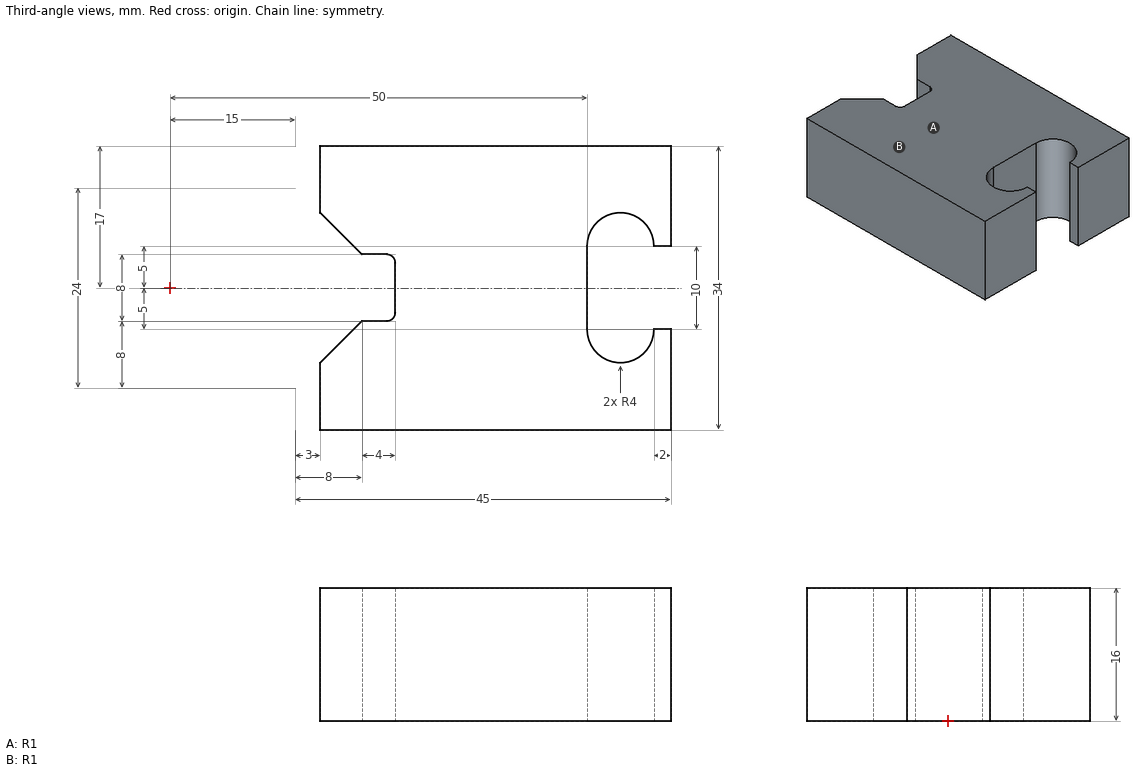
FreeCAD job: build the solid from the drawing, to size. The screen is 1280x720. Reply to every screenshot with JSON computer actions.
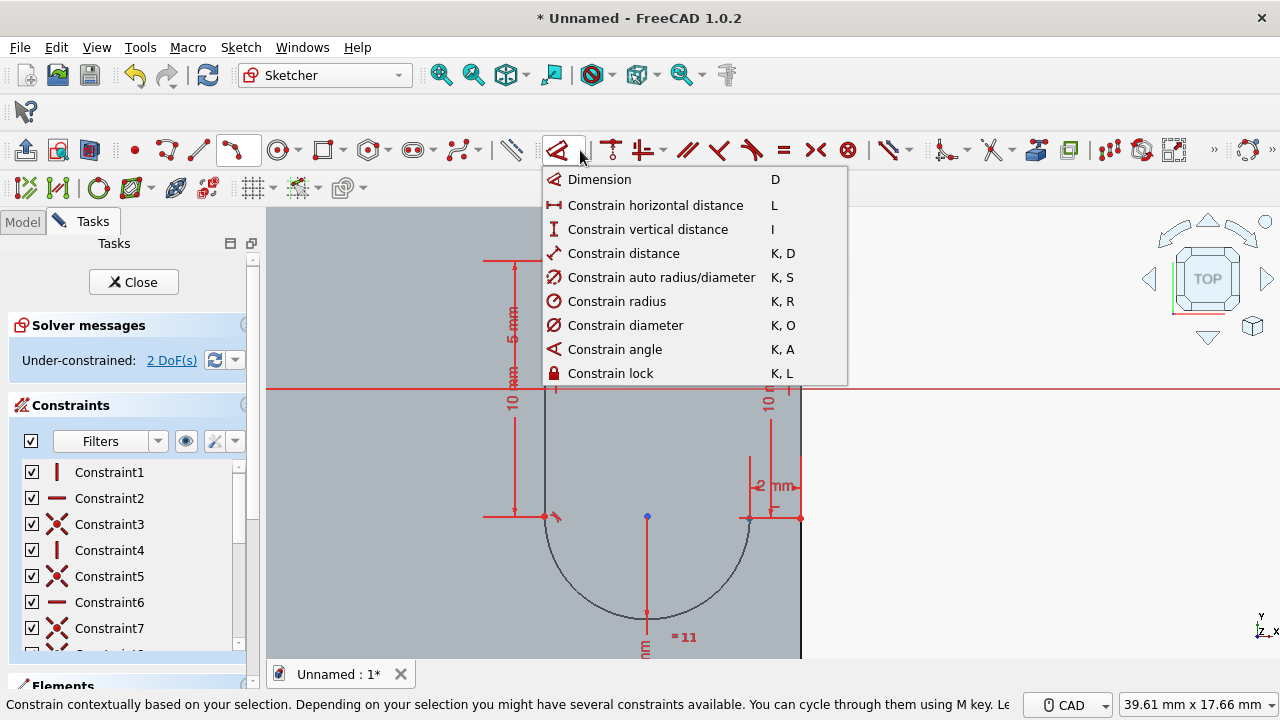
{"action": "left_click", "coordinate": [695, 229]}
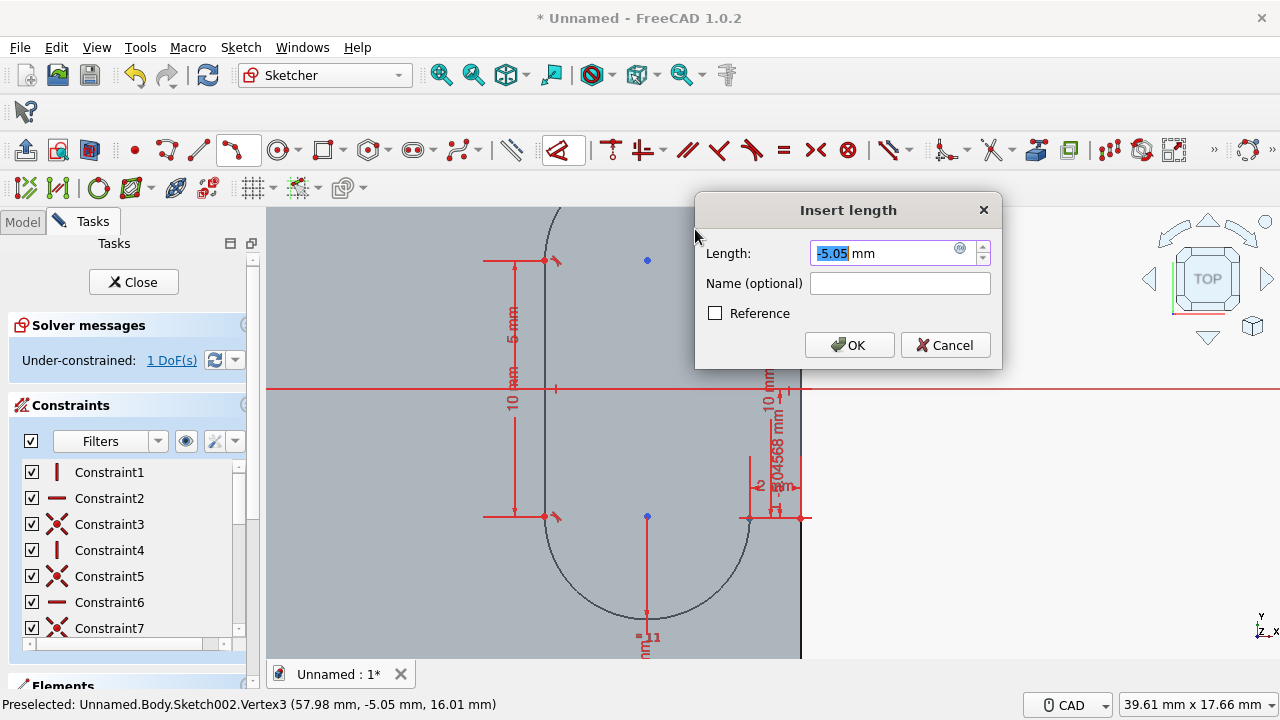
{"action": "type", "text": "-5"}
{"action": "key", "text": "Return"}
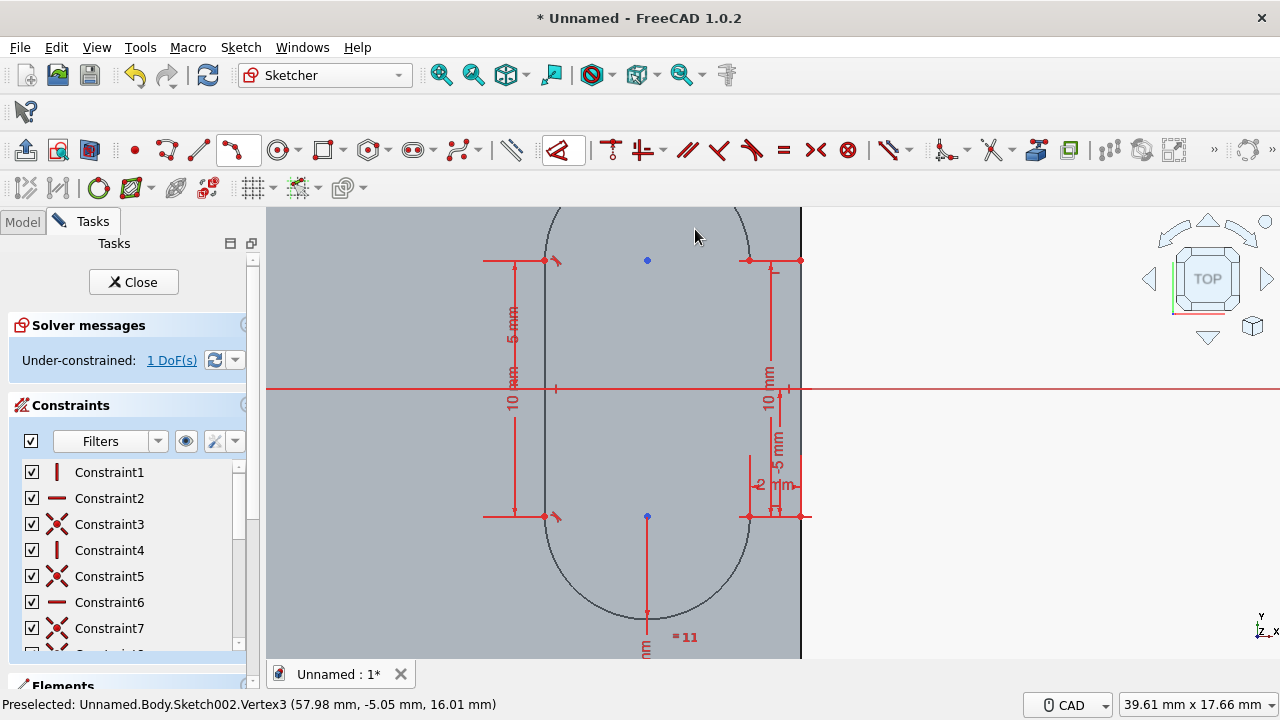
{"action": "left_click", "coordinate": [545, 261]}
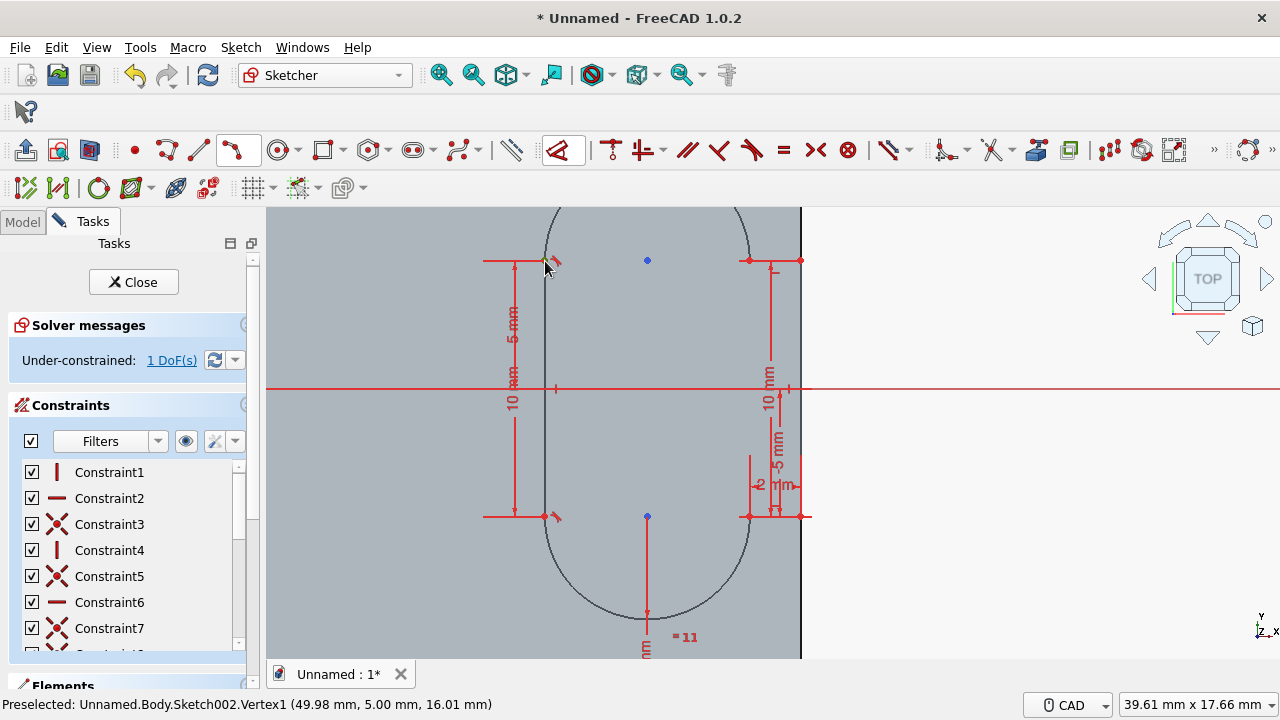
{"action": "key", "text": "l"}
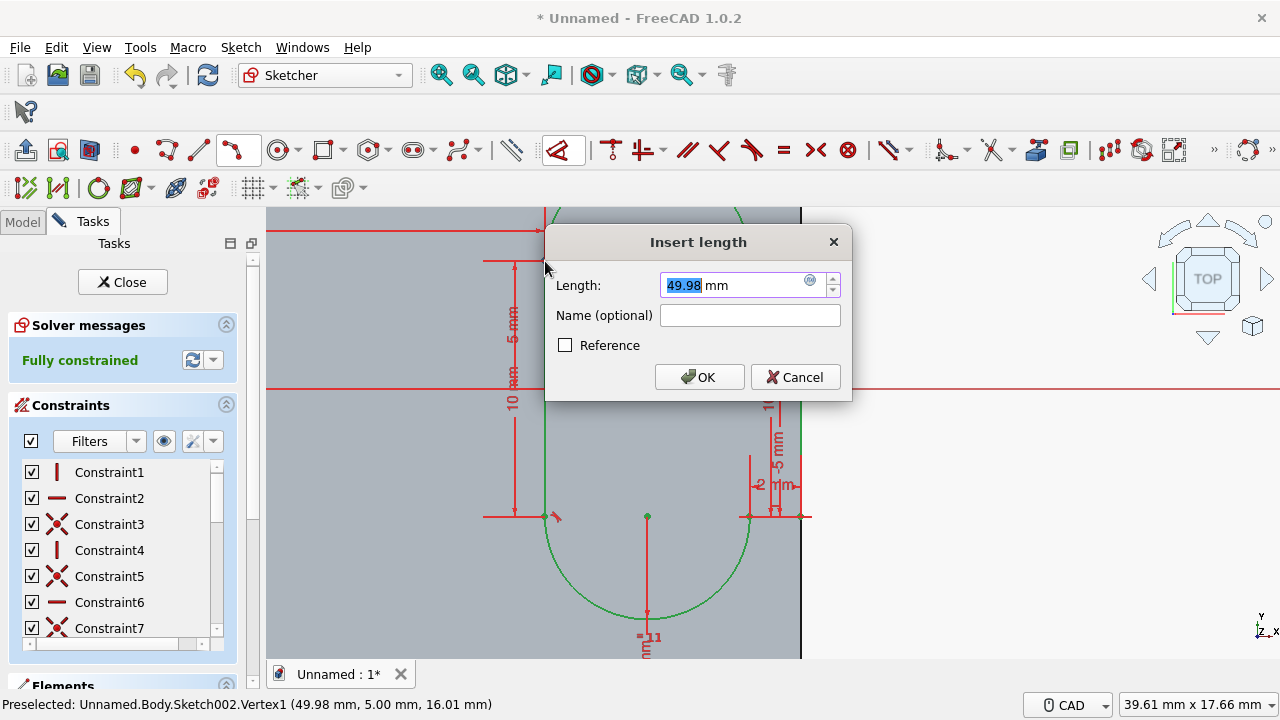
{"action": "type", "text": "50"}
{"action": "key", "text": "Return"}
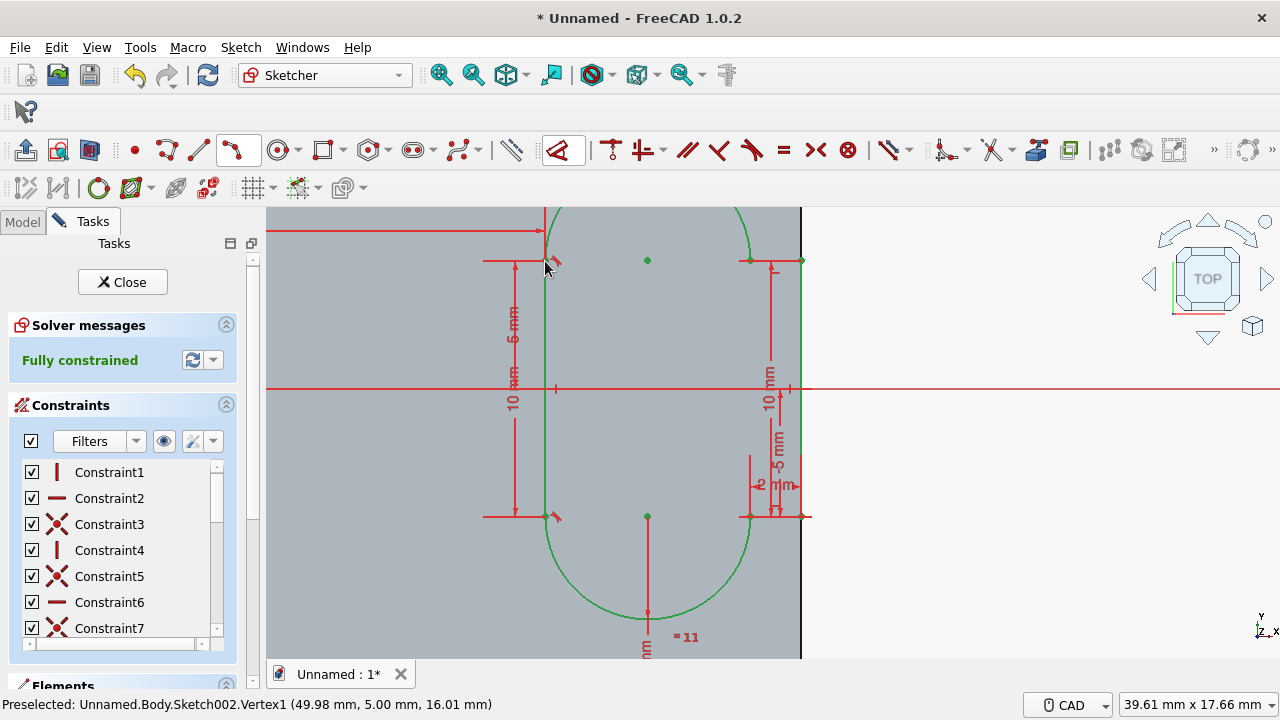
{"action": "left_click", "coordinate": [123, 282]}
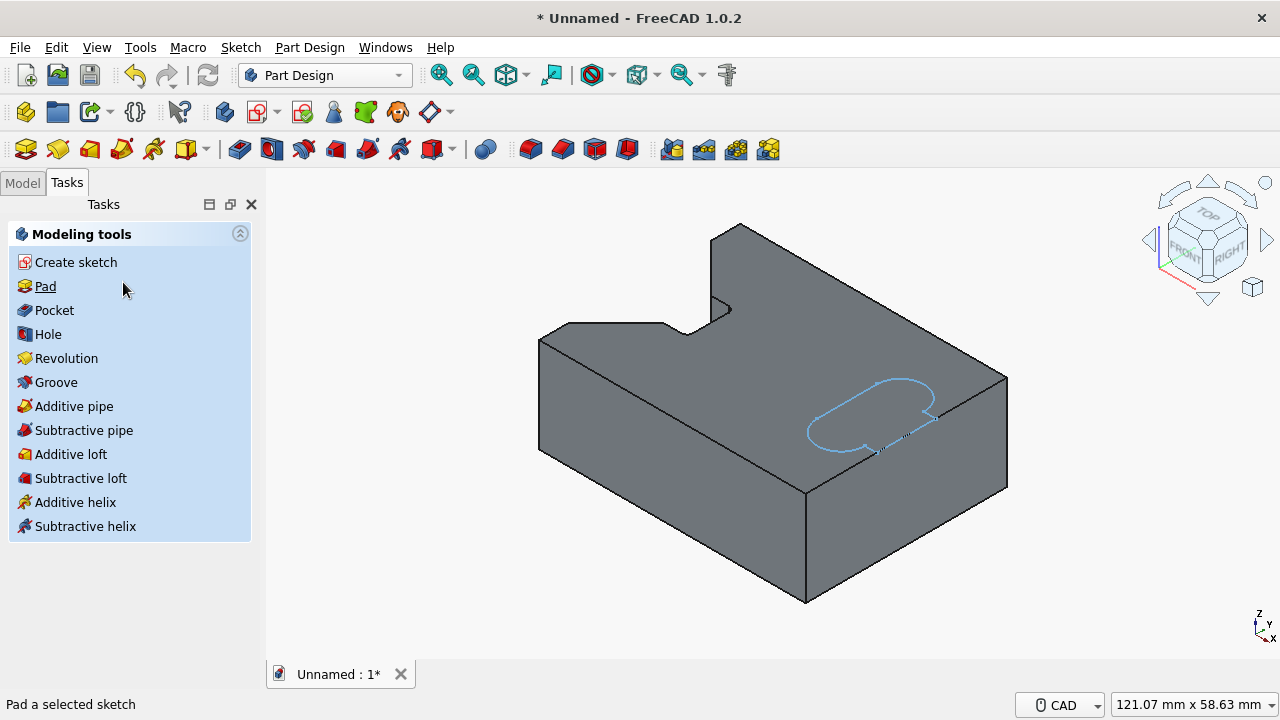
{"action": "left_click", "coordinate": [240, 150]}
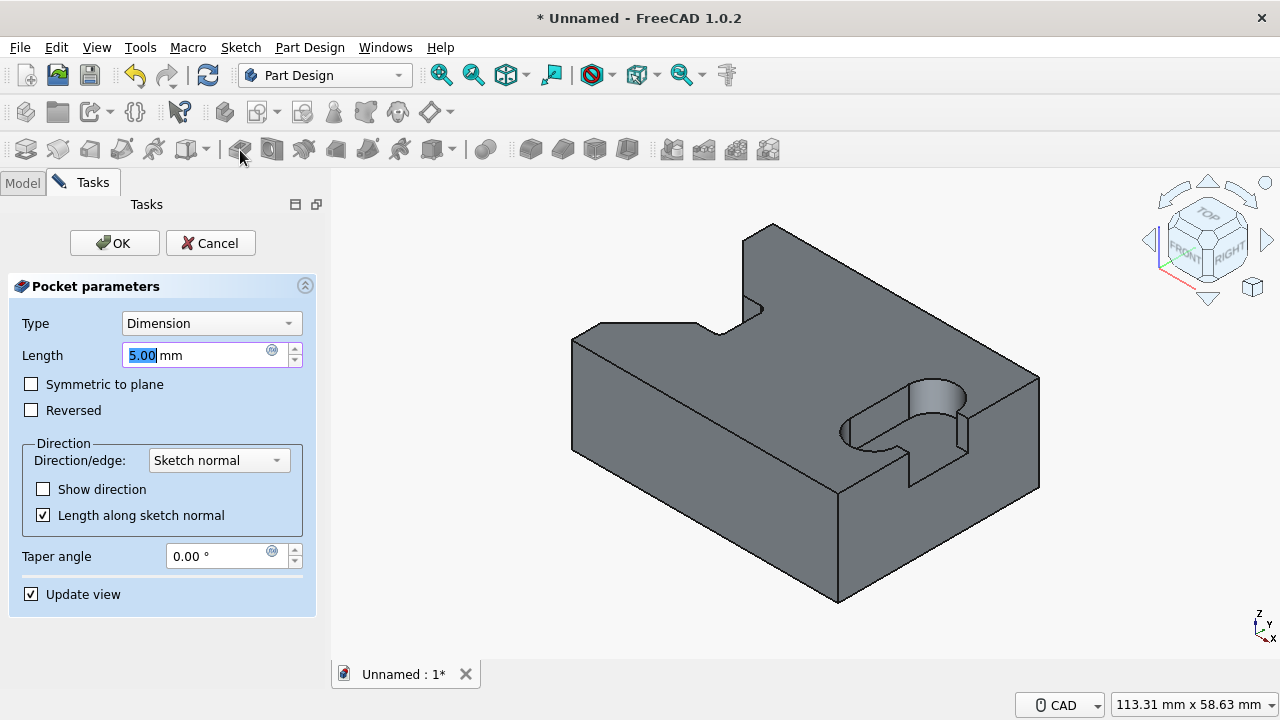
{"action": "left_click", "coordinate": [212, 324]}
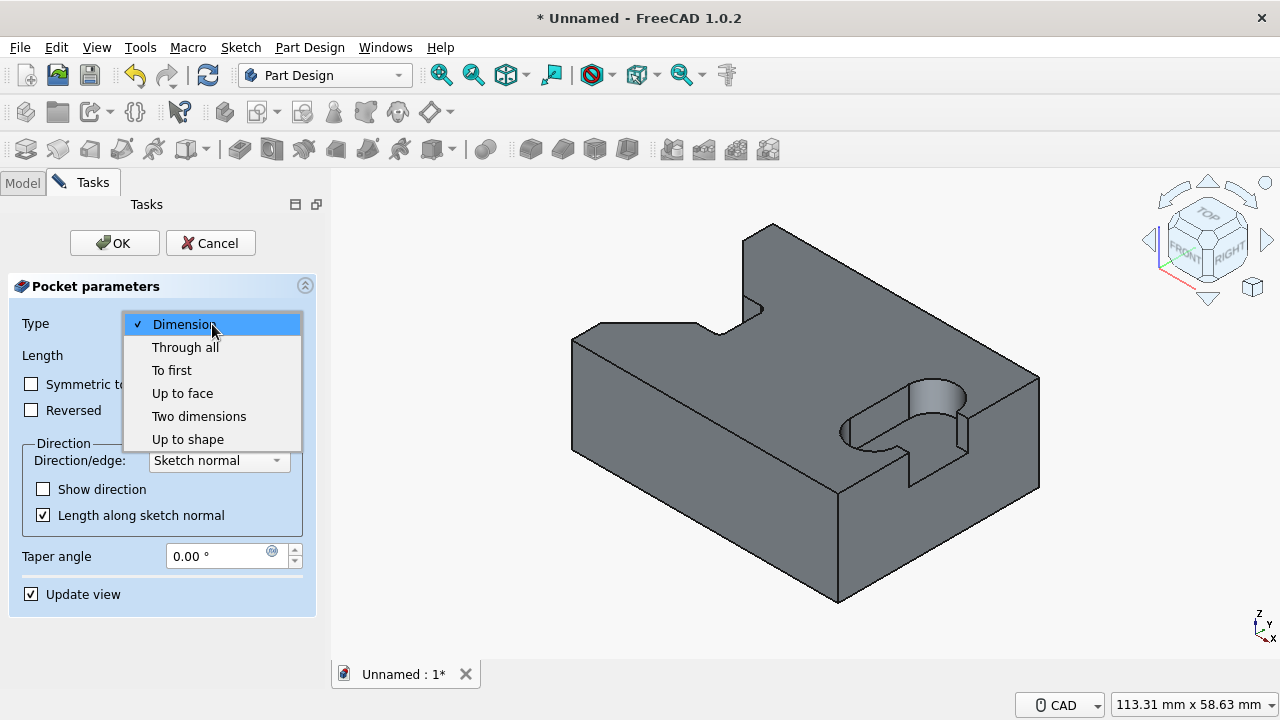
{"action": "left_click", "coordinate": [212, 348]}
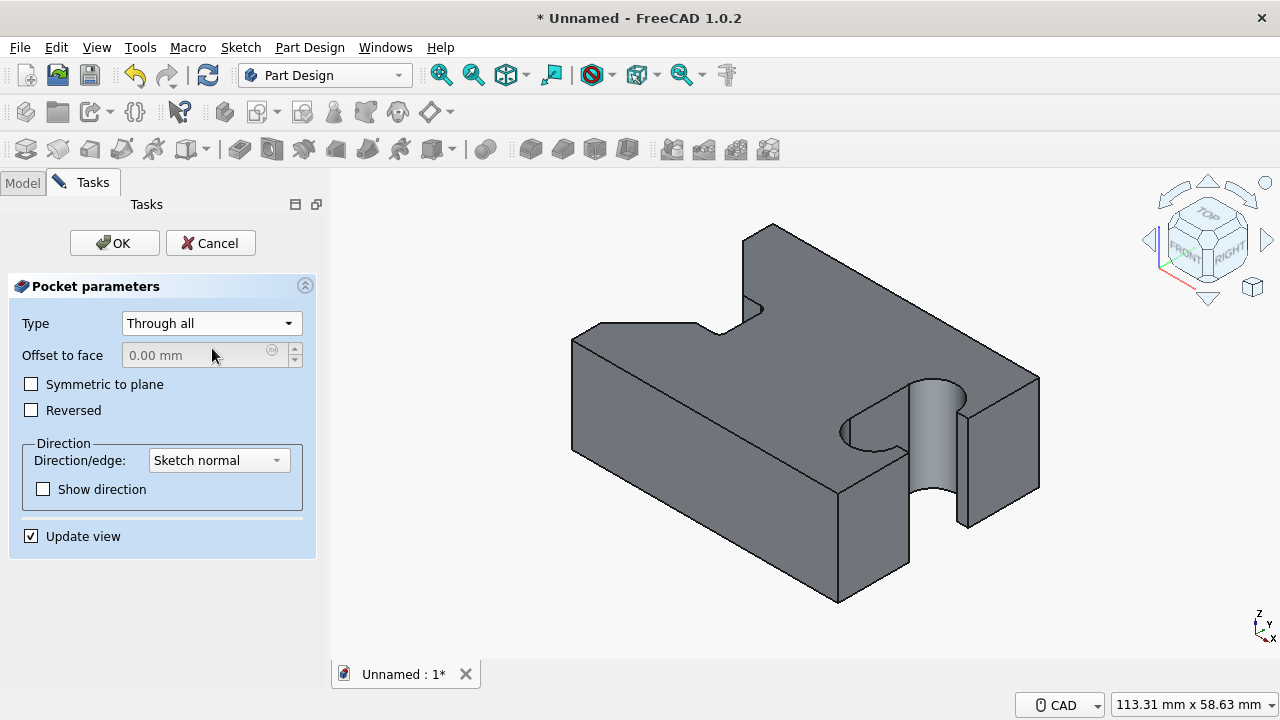
{"action": "left_click", "coordinate": [115, 243]}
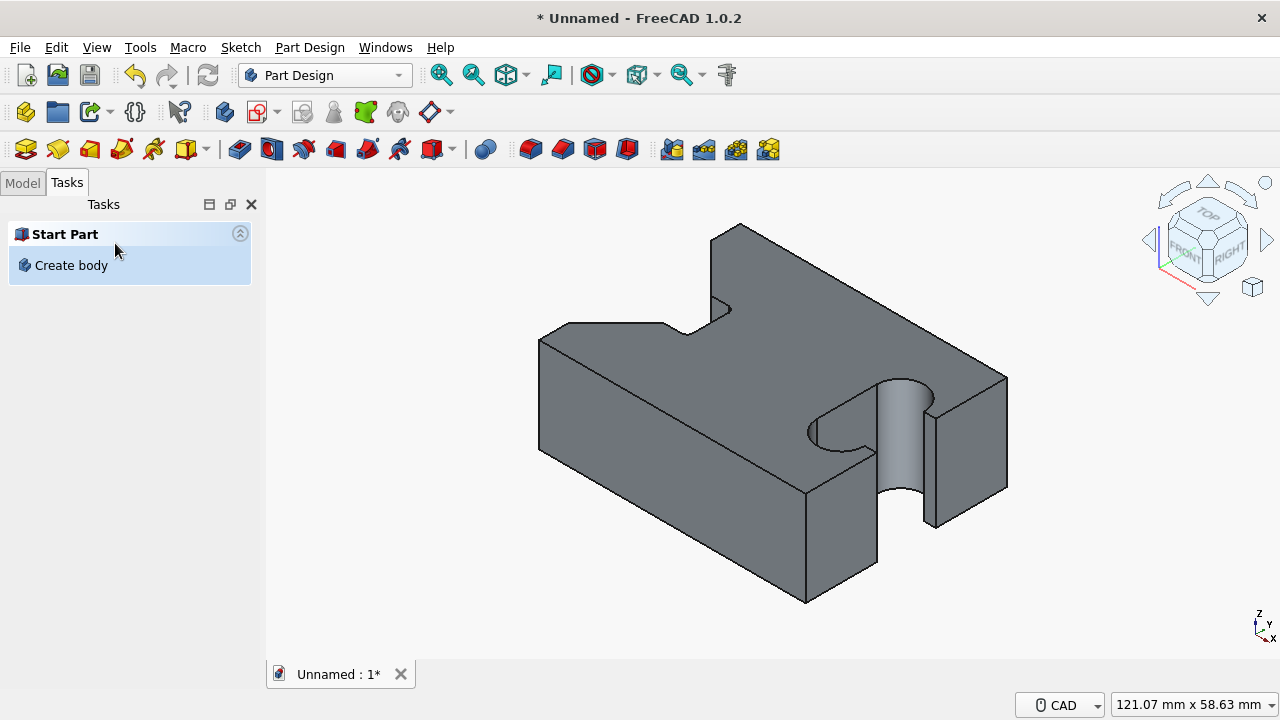
{"action": "left_click", "coordinate": [802, 341]}